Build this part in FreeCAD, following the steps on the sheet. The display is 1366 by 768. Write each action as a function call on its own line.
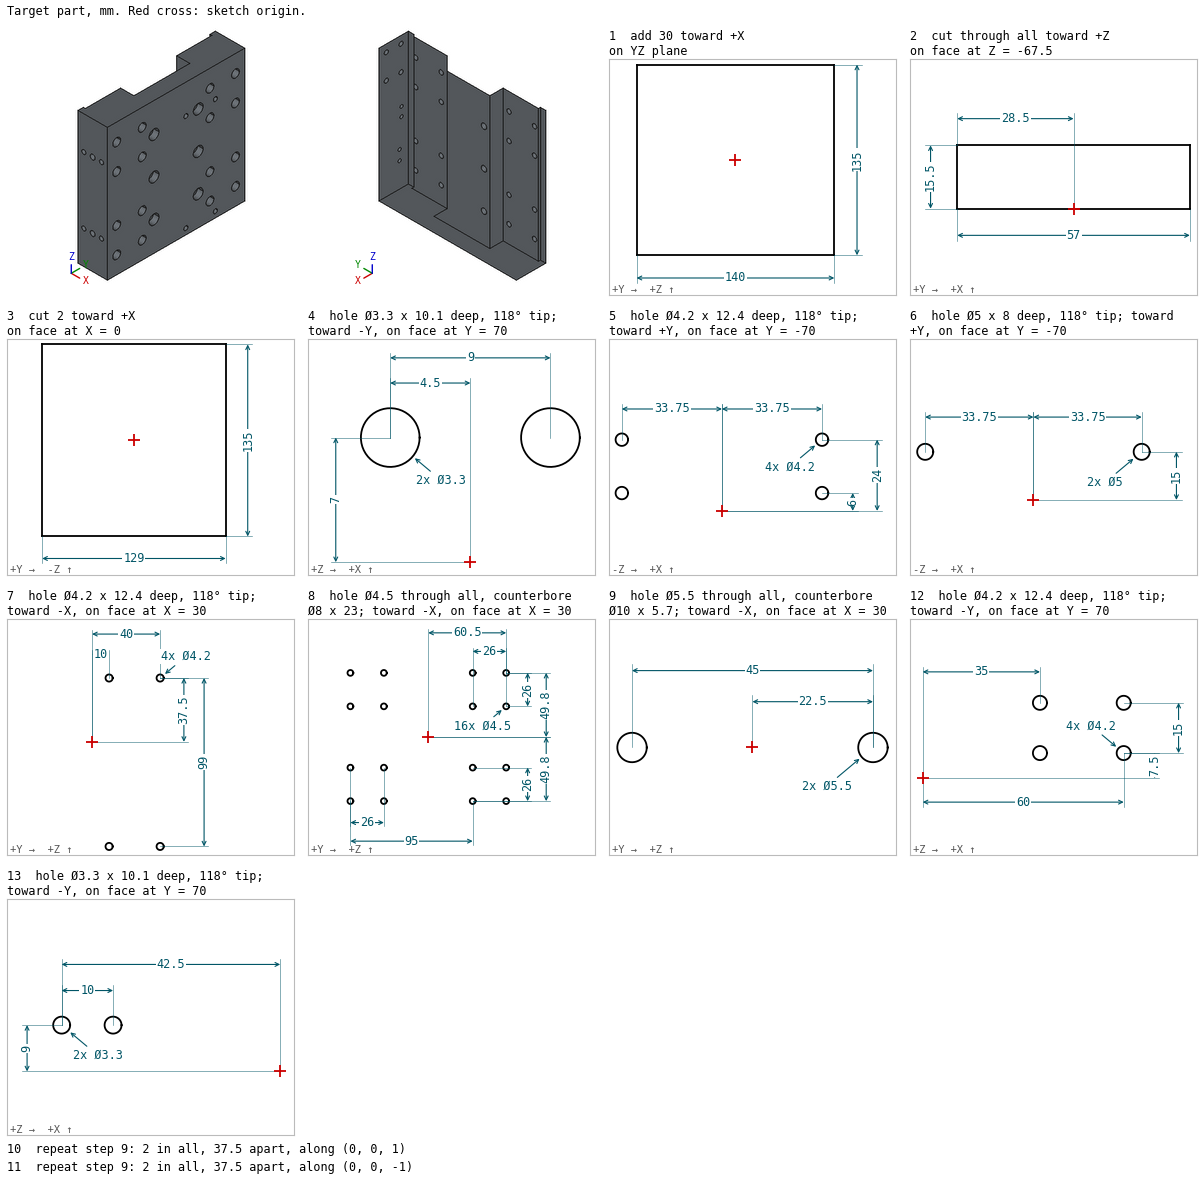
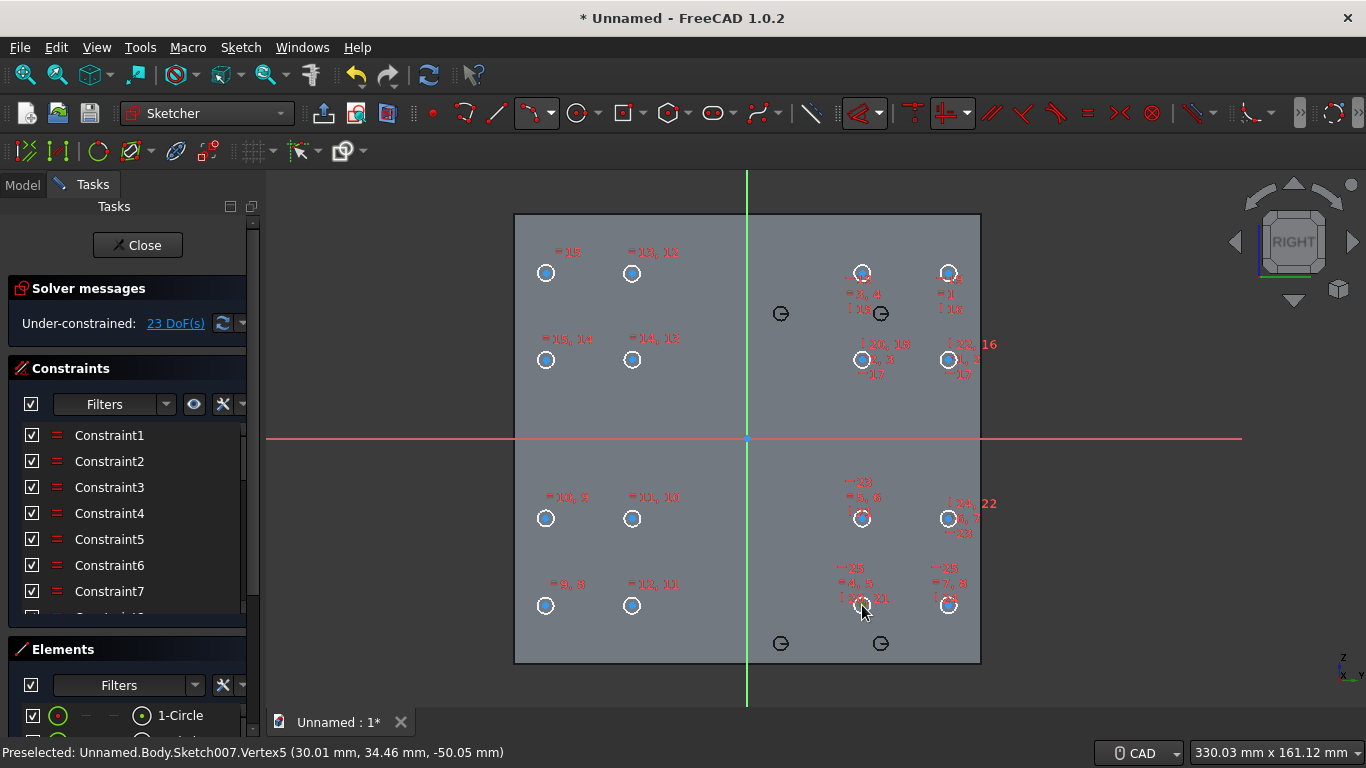
click(546, 606)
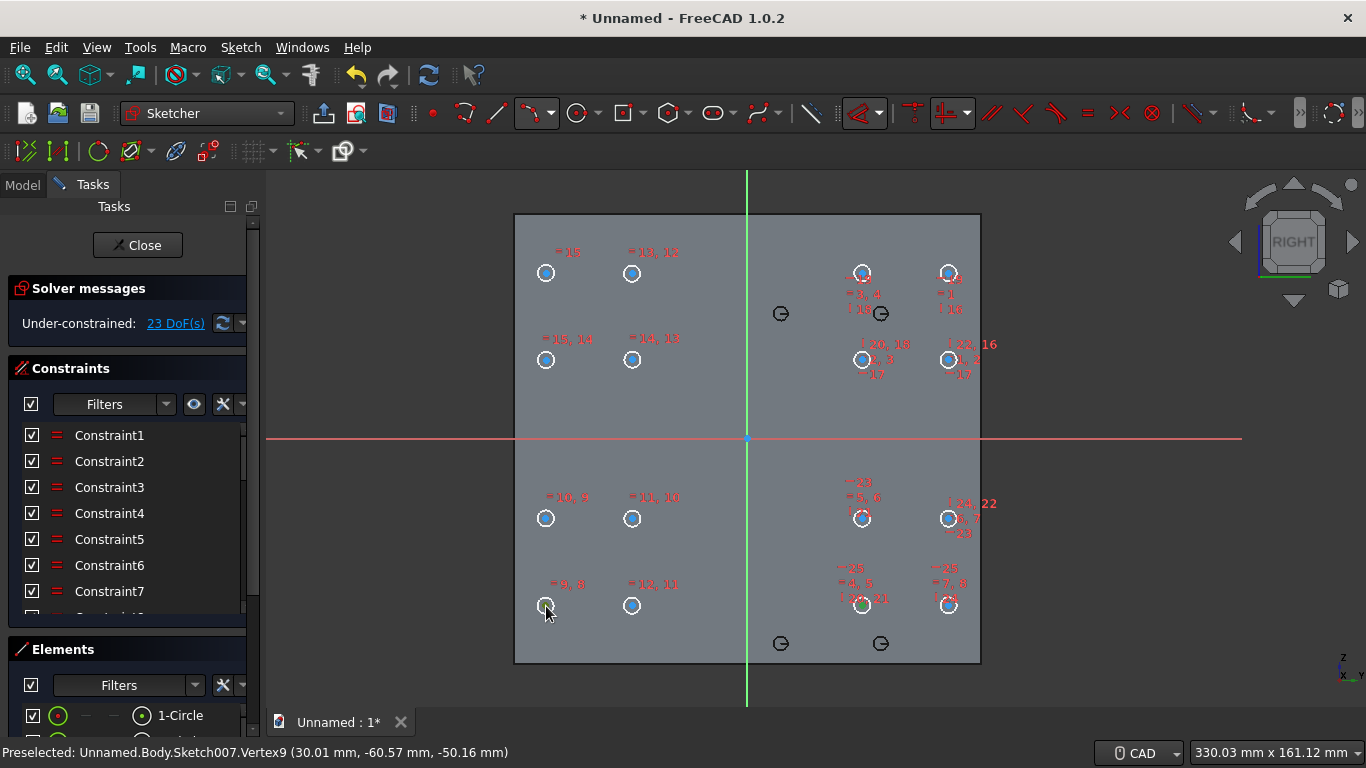
click(970, 114)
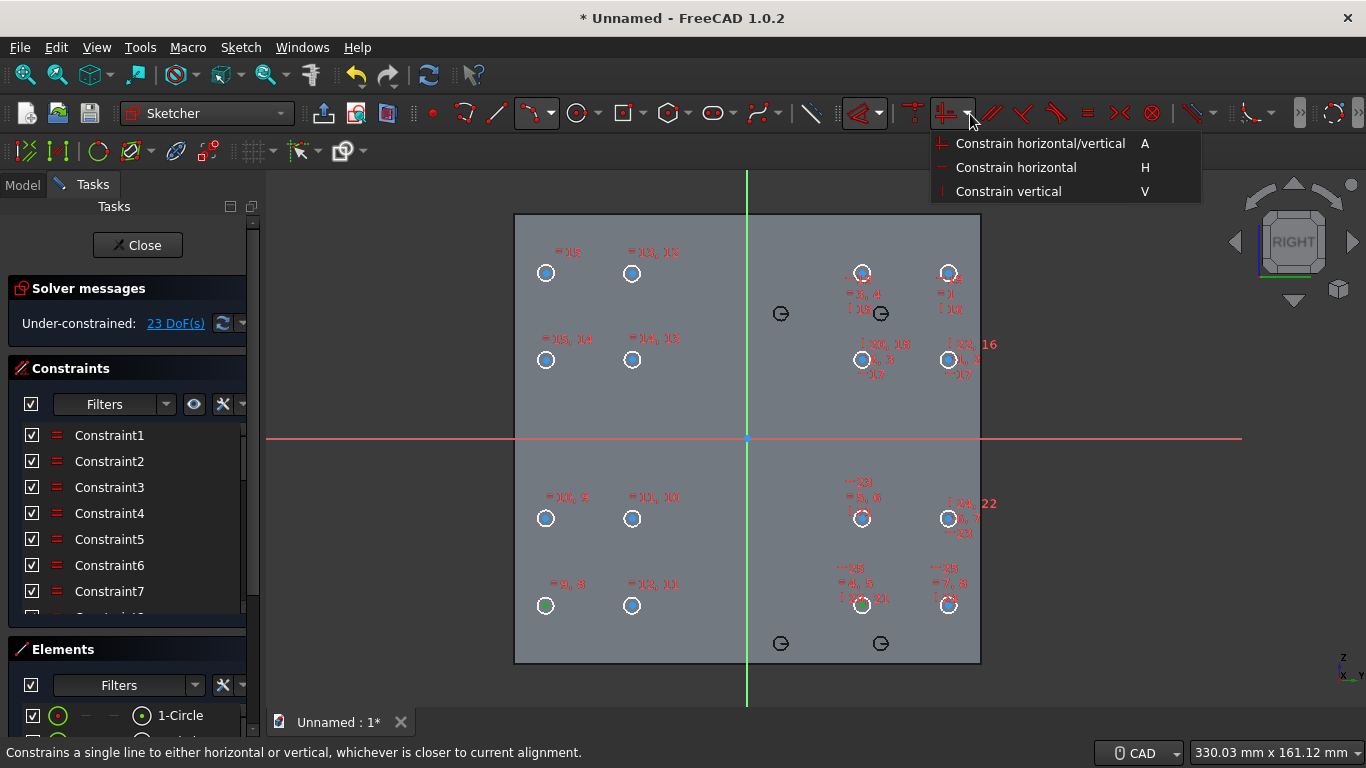
click(1066, 167)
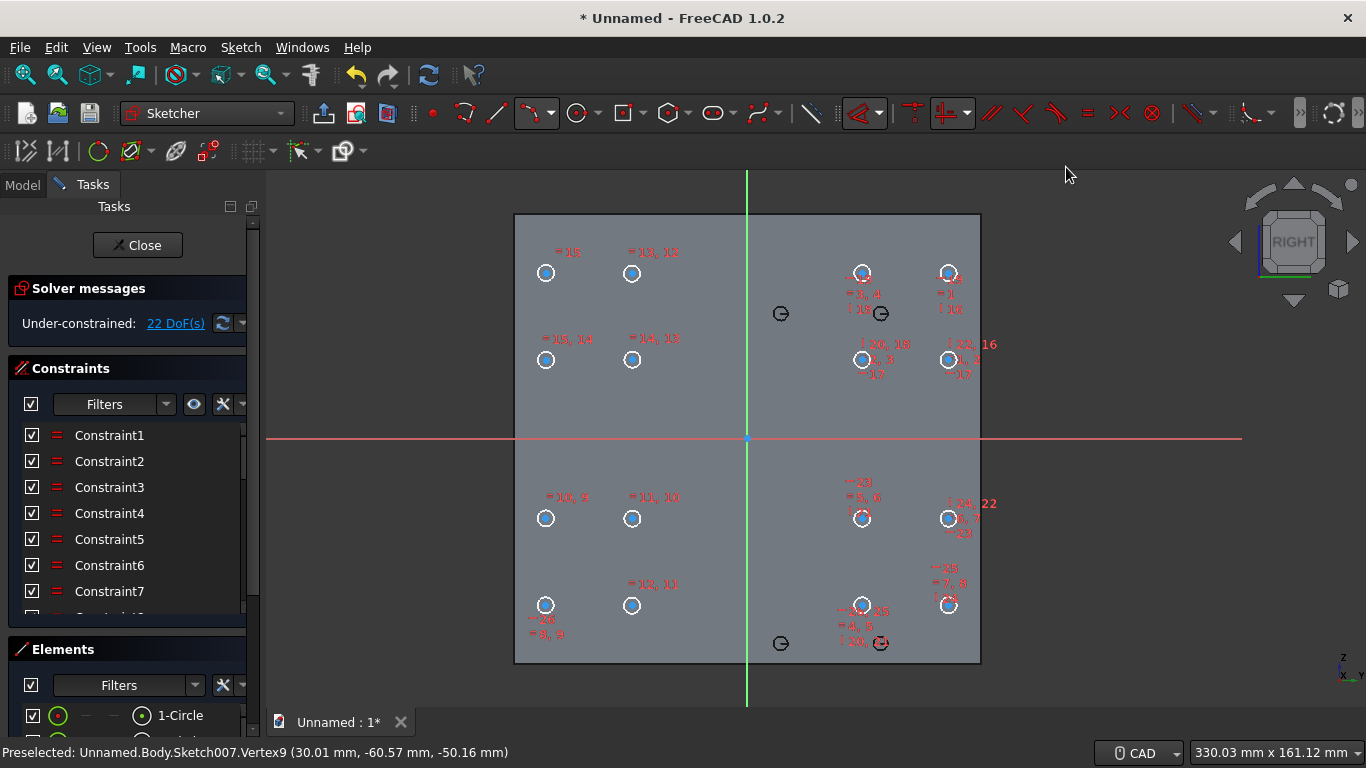
click(546, 605)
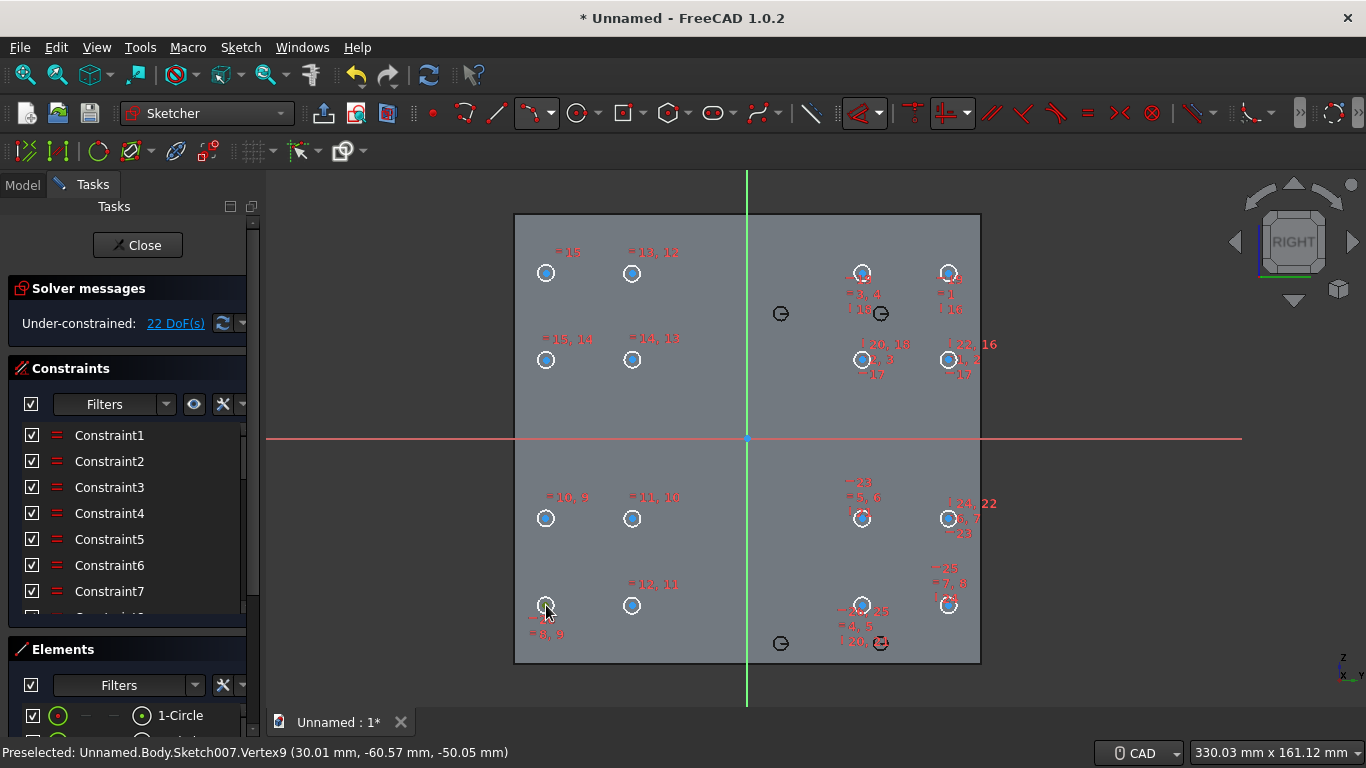
click(546, 518)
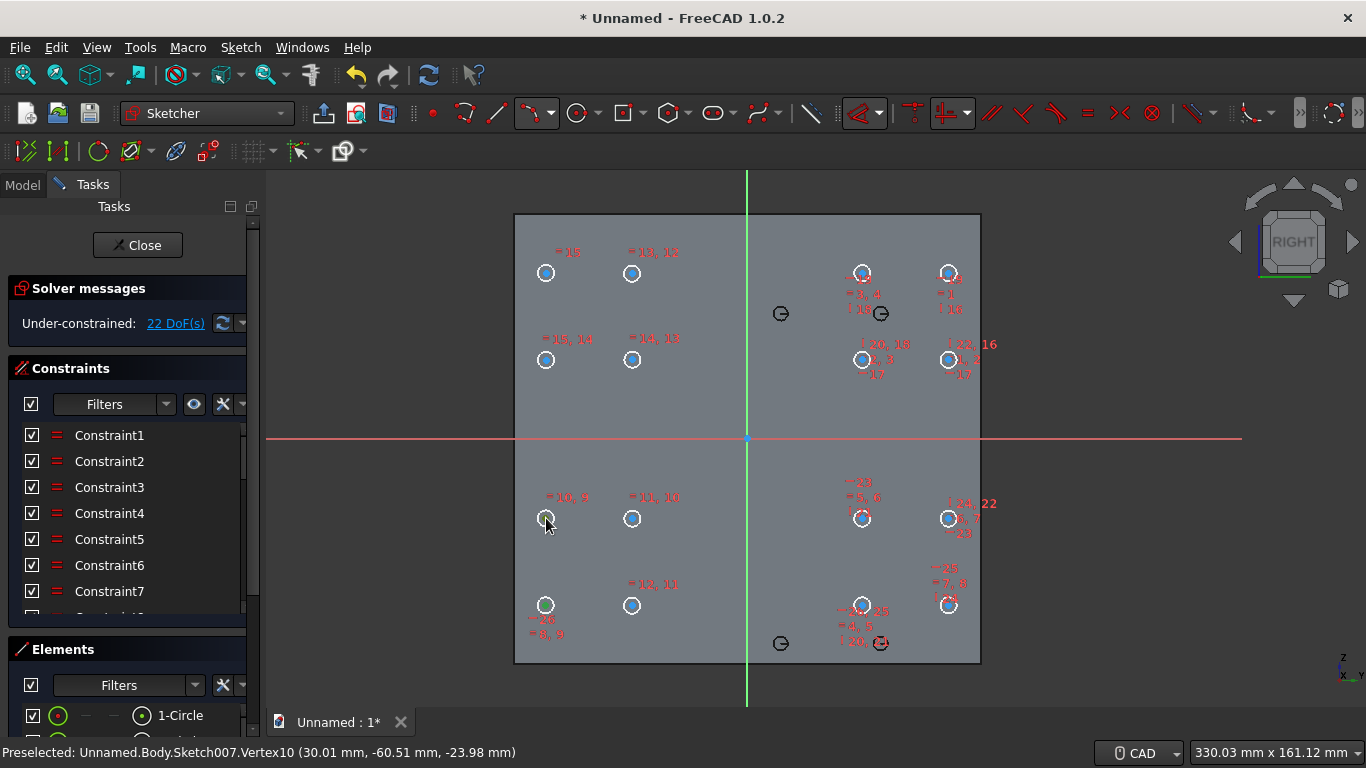
key(v)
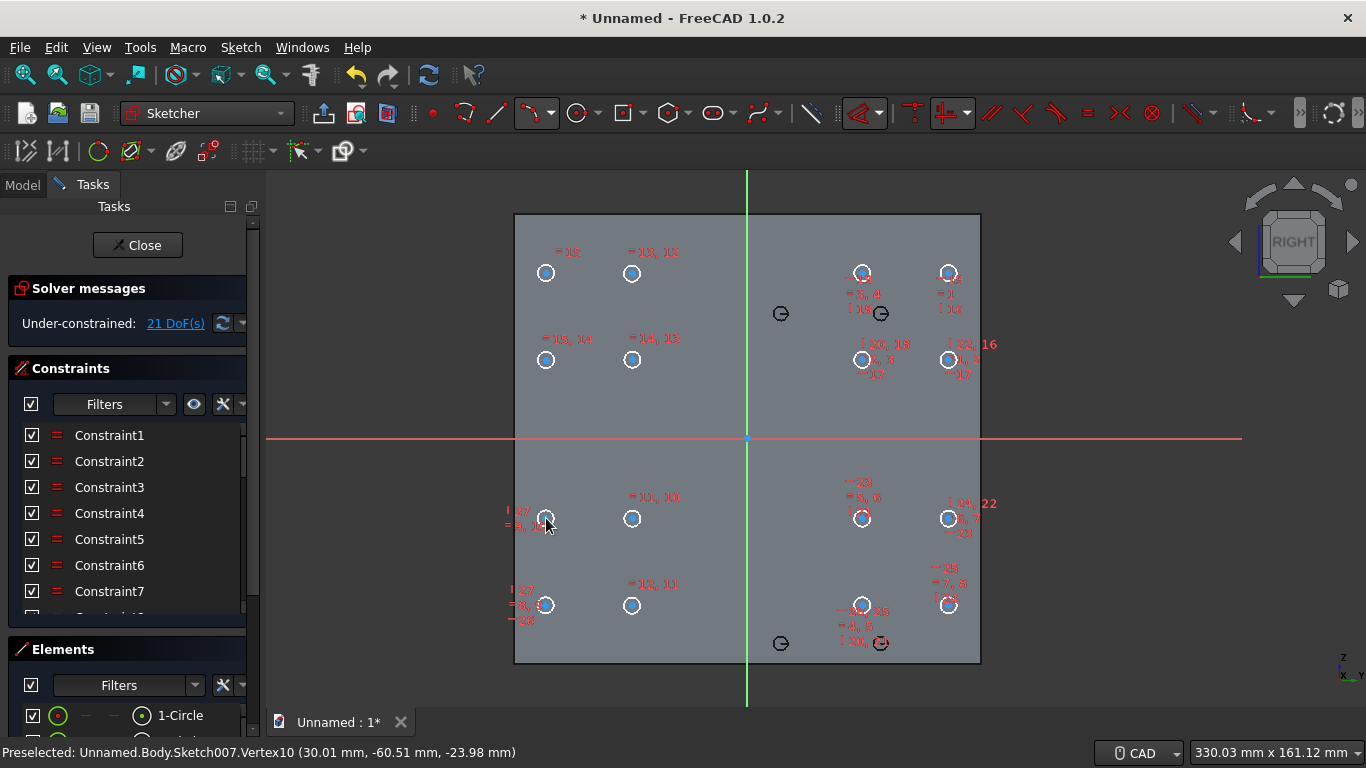
click(862, 519)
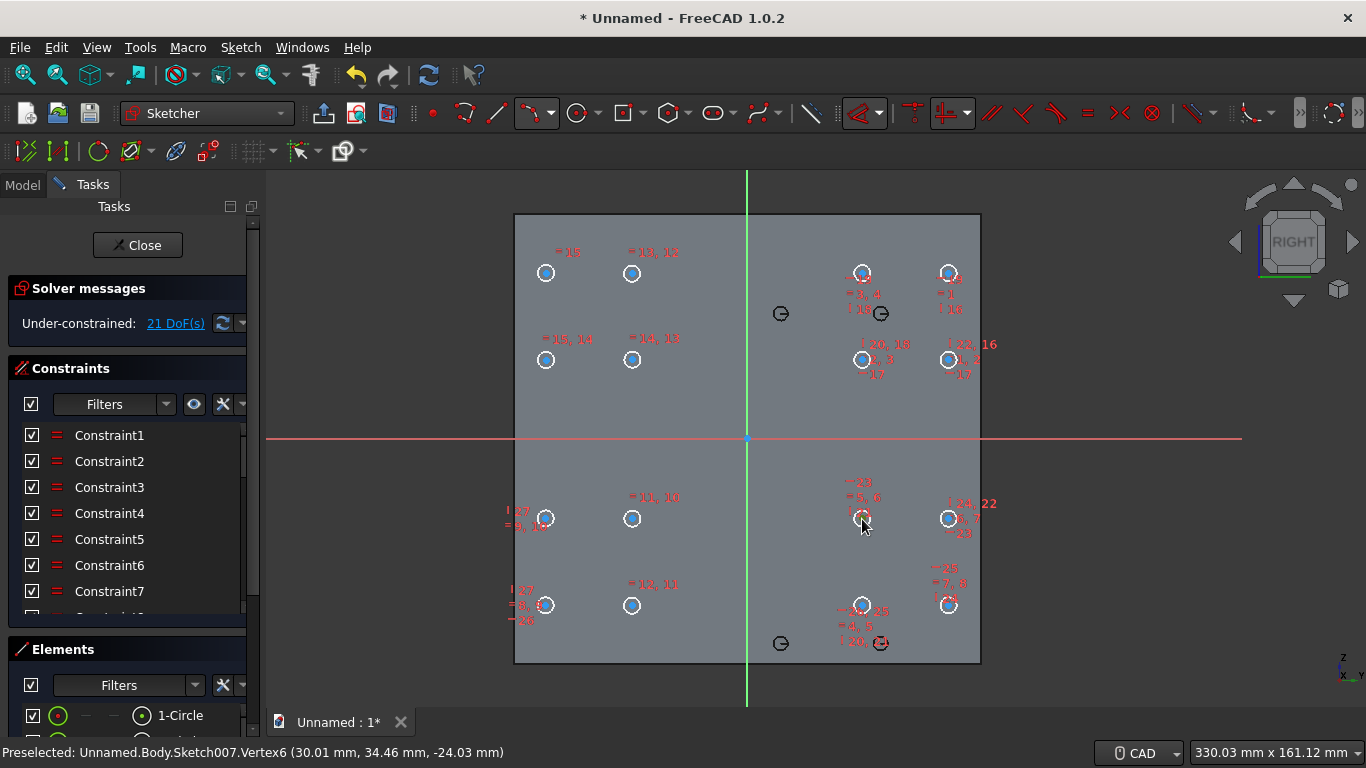
click(548, 520)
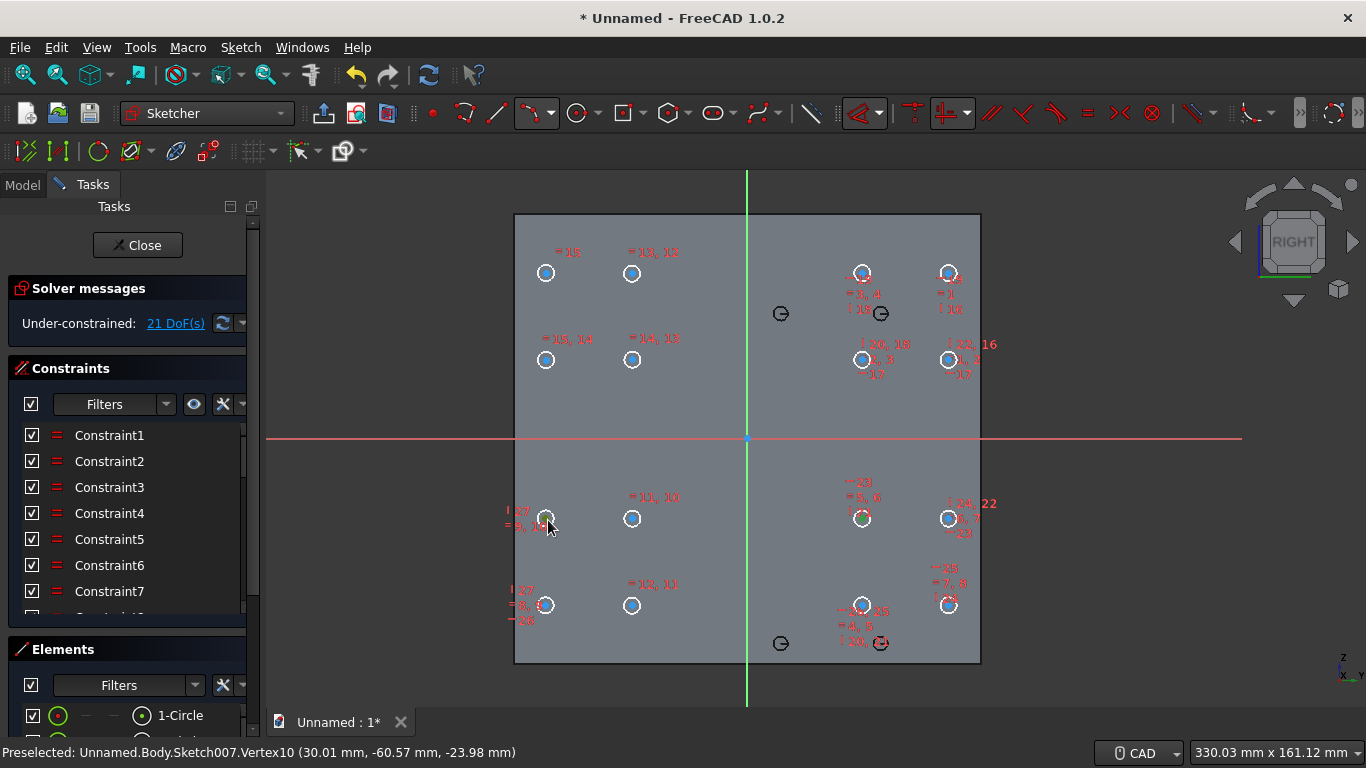
click(970, 114)